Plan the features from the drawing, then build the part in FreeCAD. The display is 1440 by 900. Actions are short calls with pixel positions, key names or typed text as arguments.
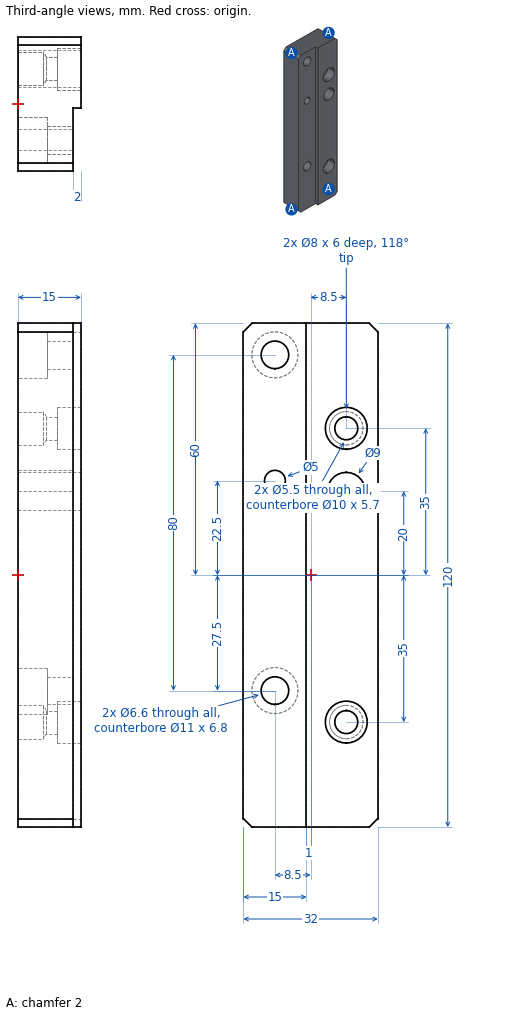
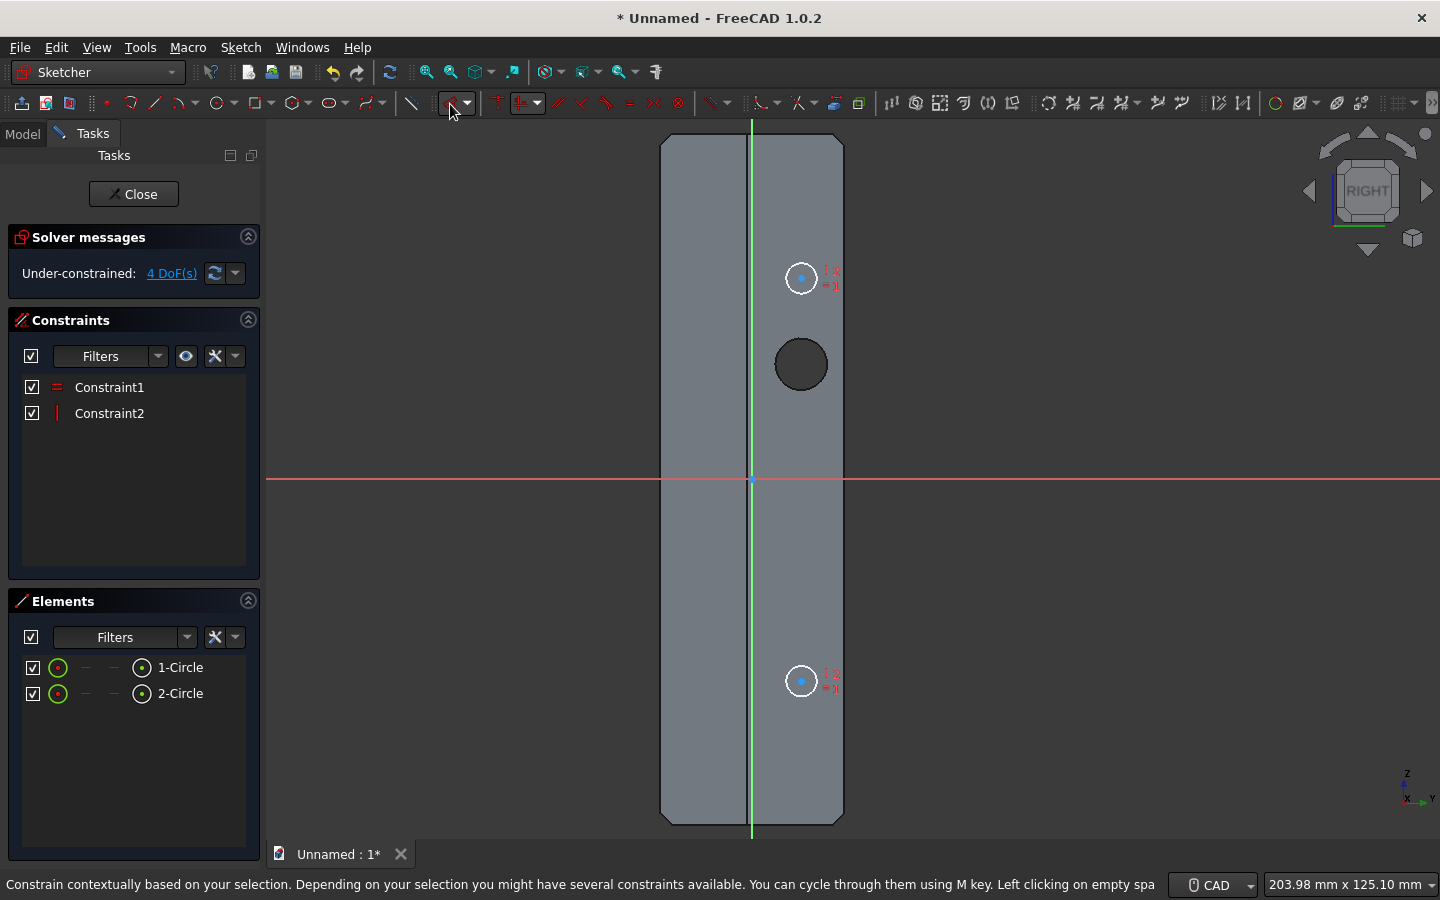
scroll(812, 268, up, 2)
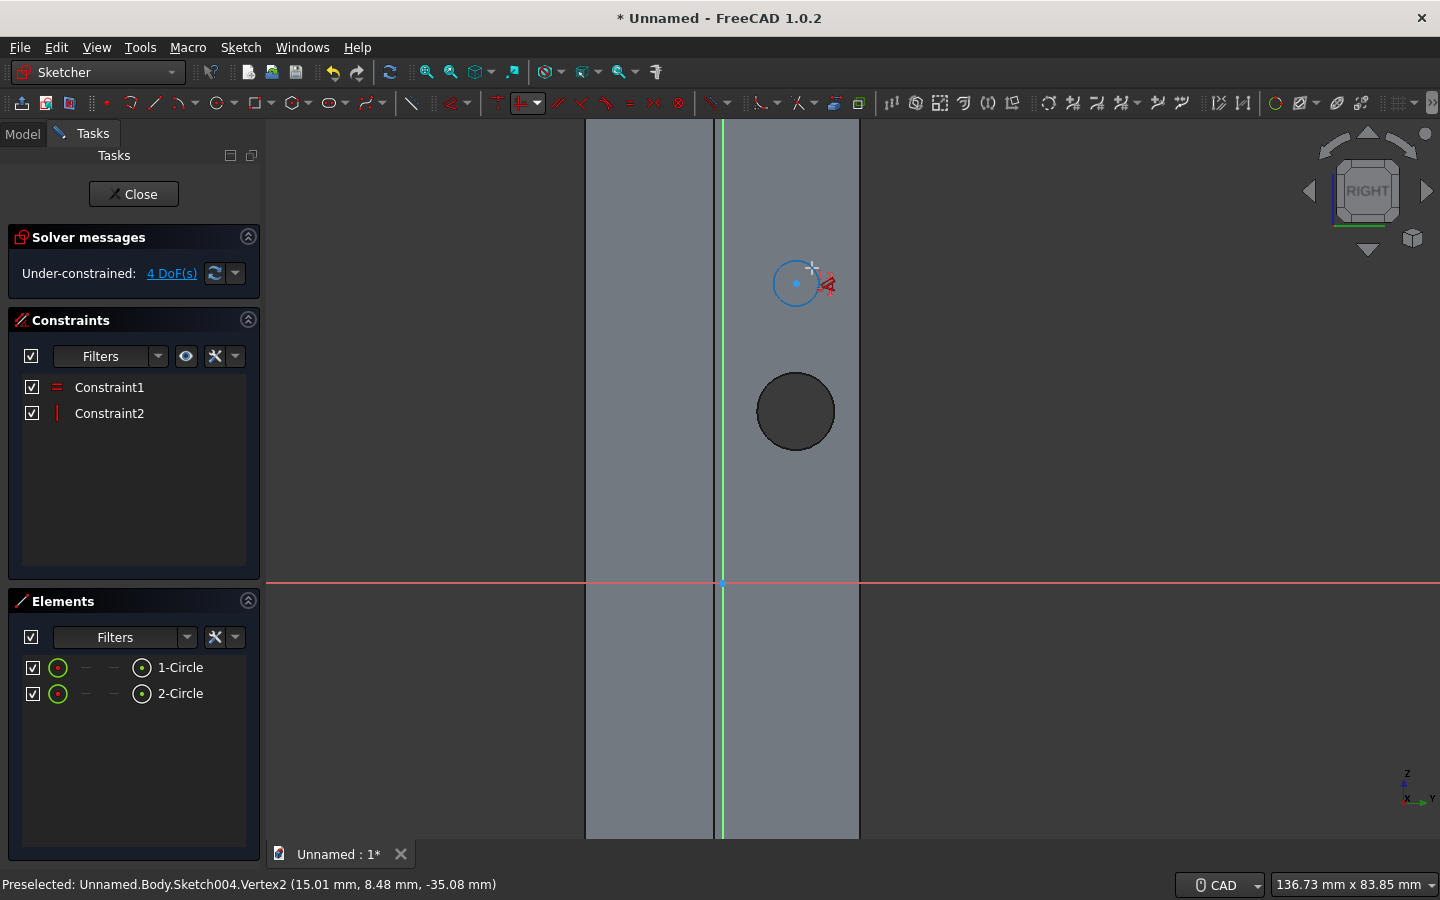
click(812, 267)
click(834, 244)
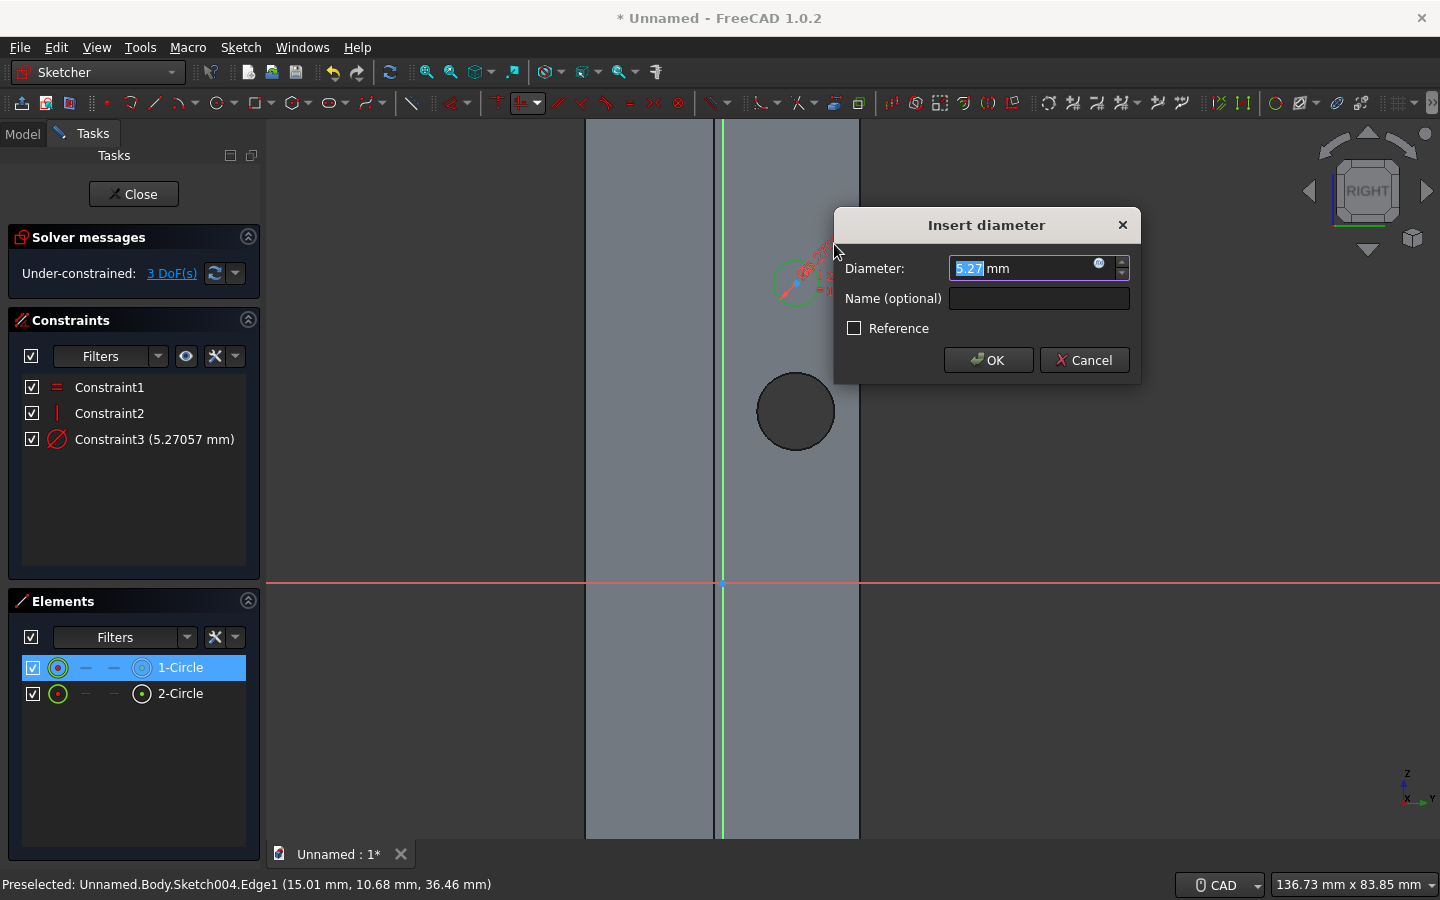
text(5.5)
key(Return)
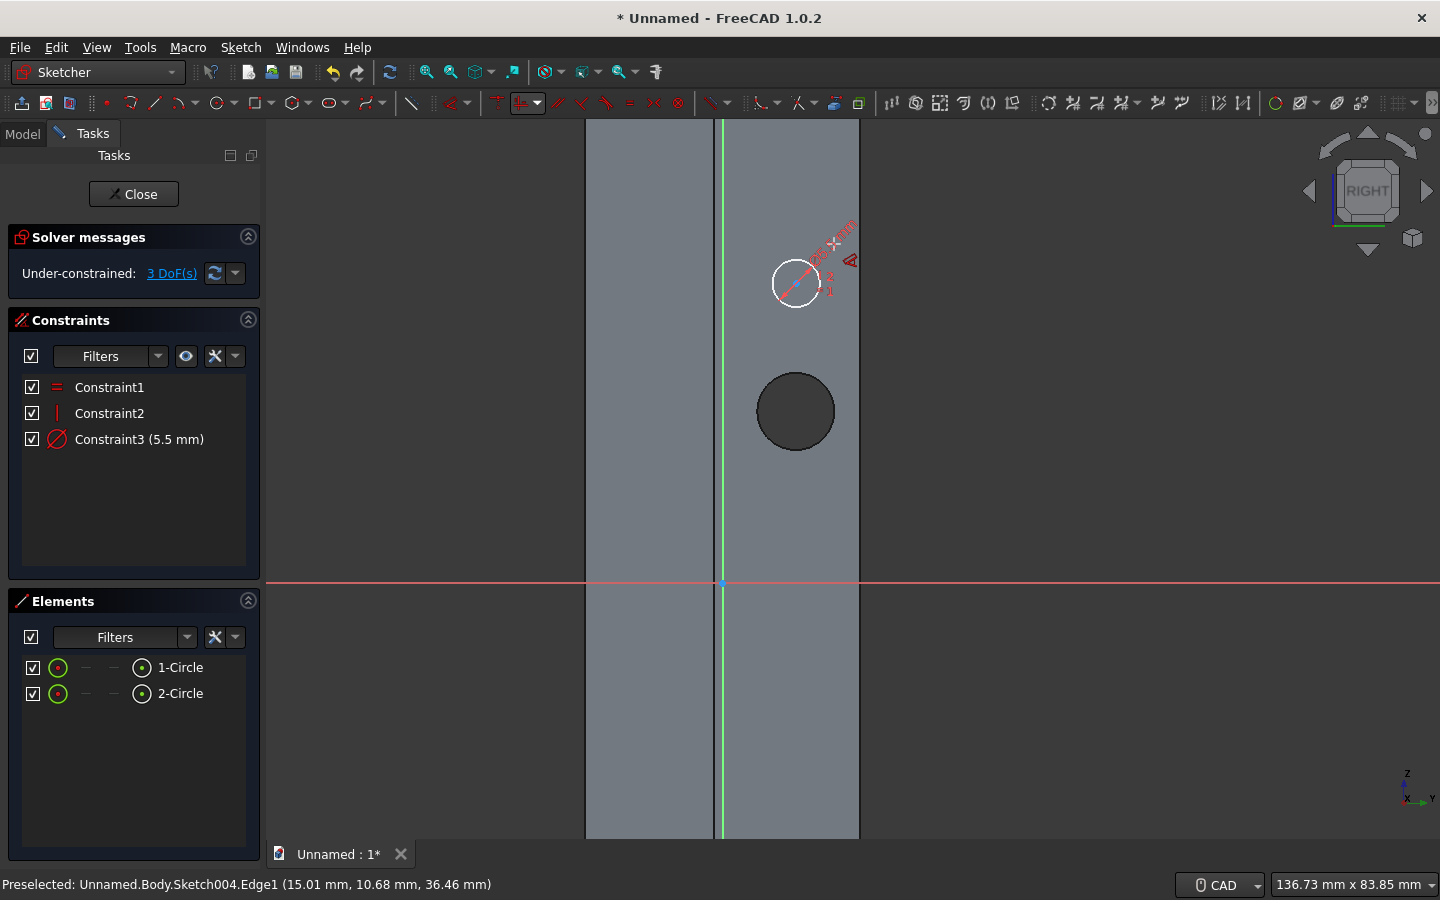
click(796, 283)
click(689, 433)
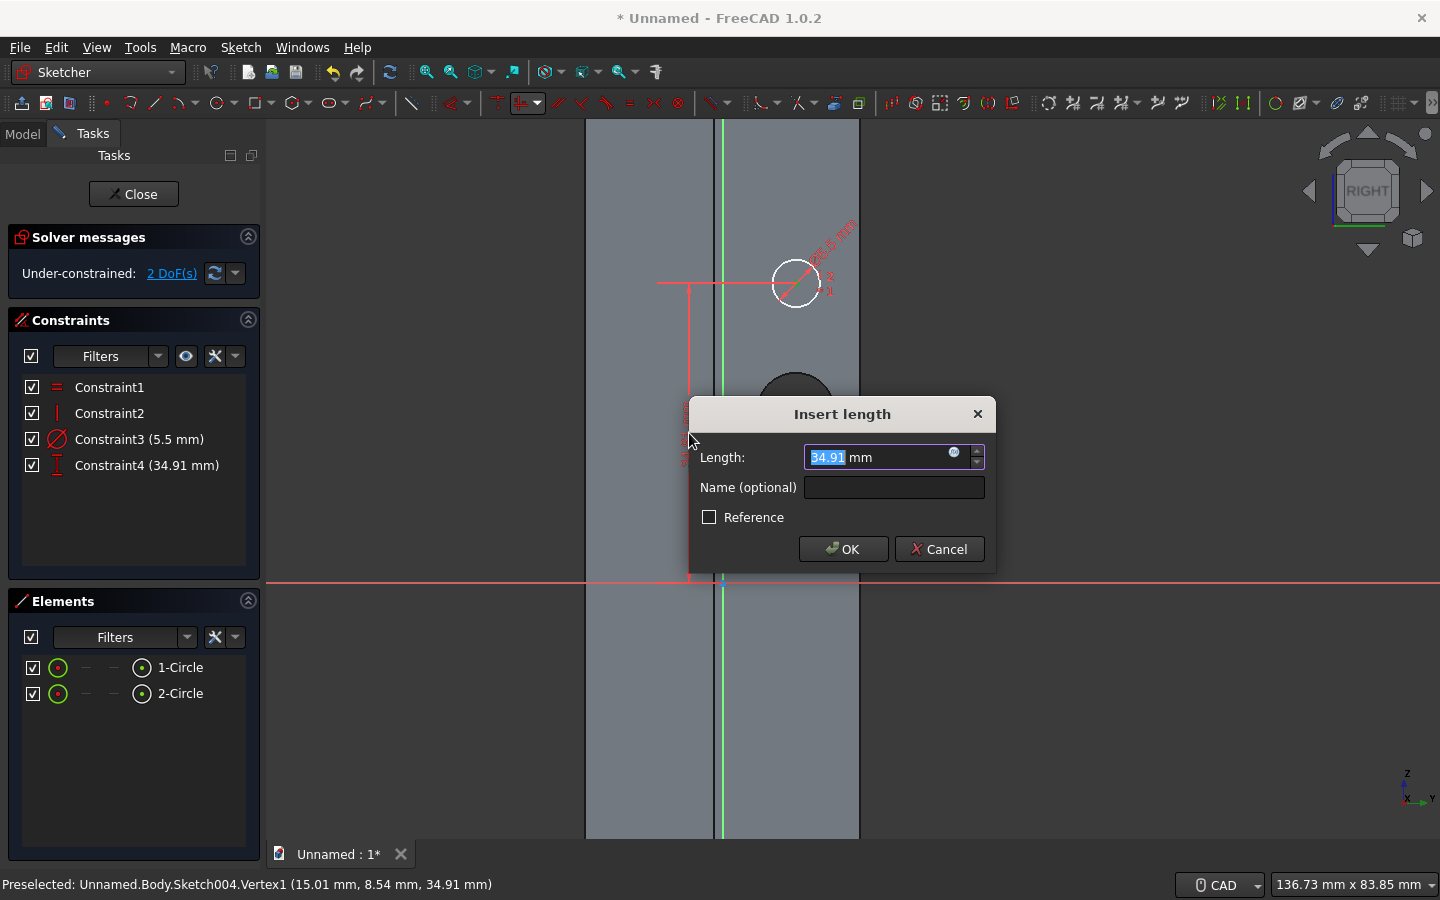
text(35)
key(Return)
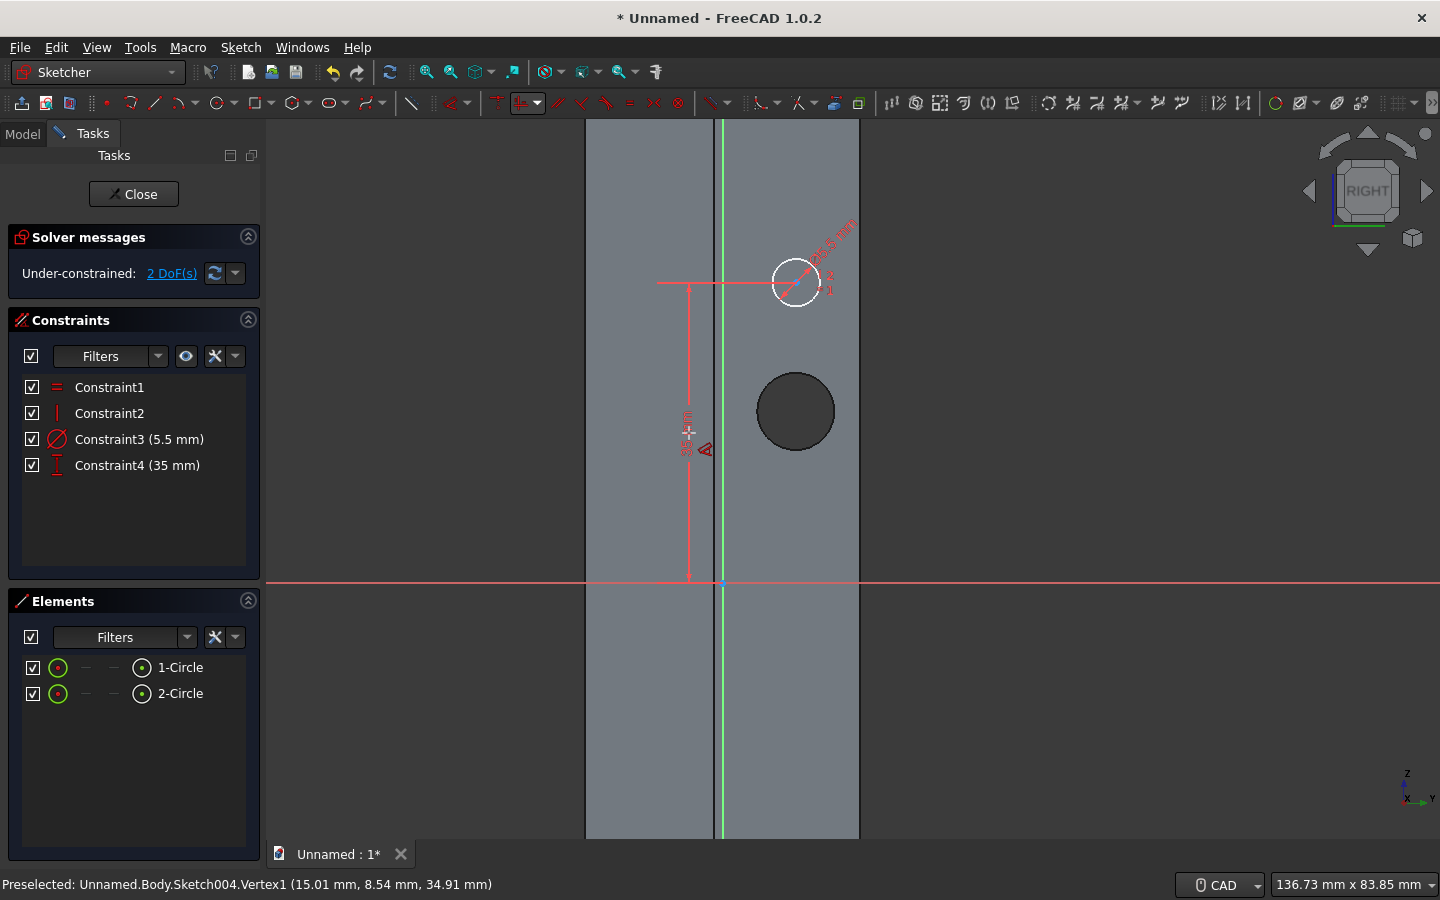
scroll(812, 267, down, 2)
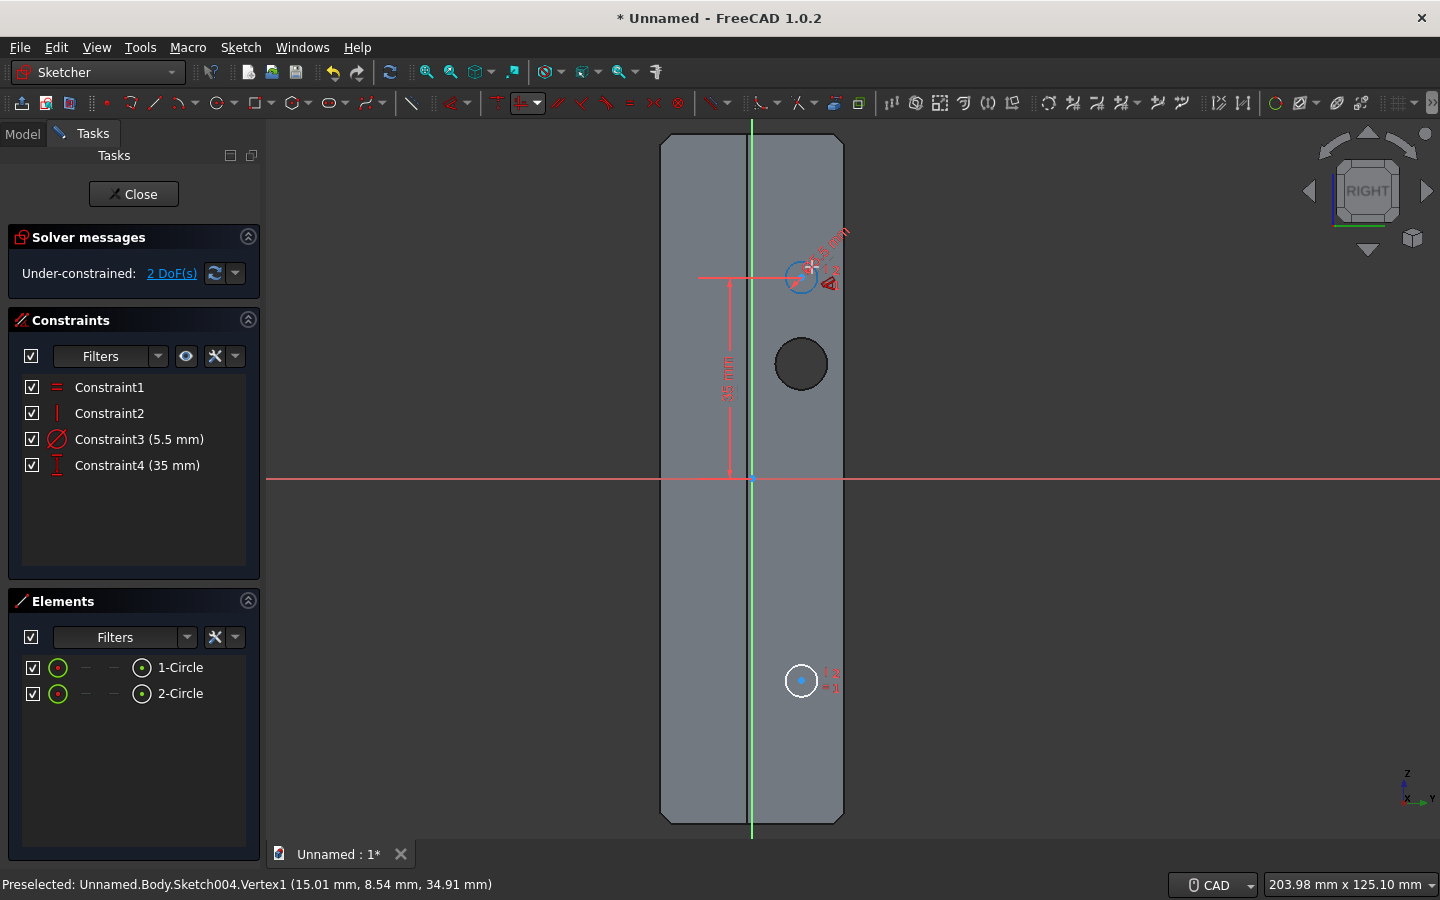
click(802, 681)
click(718, 580)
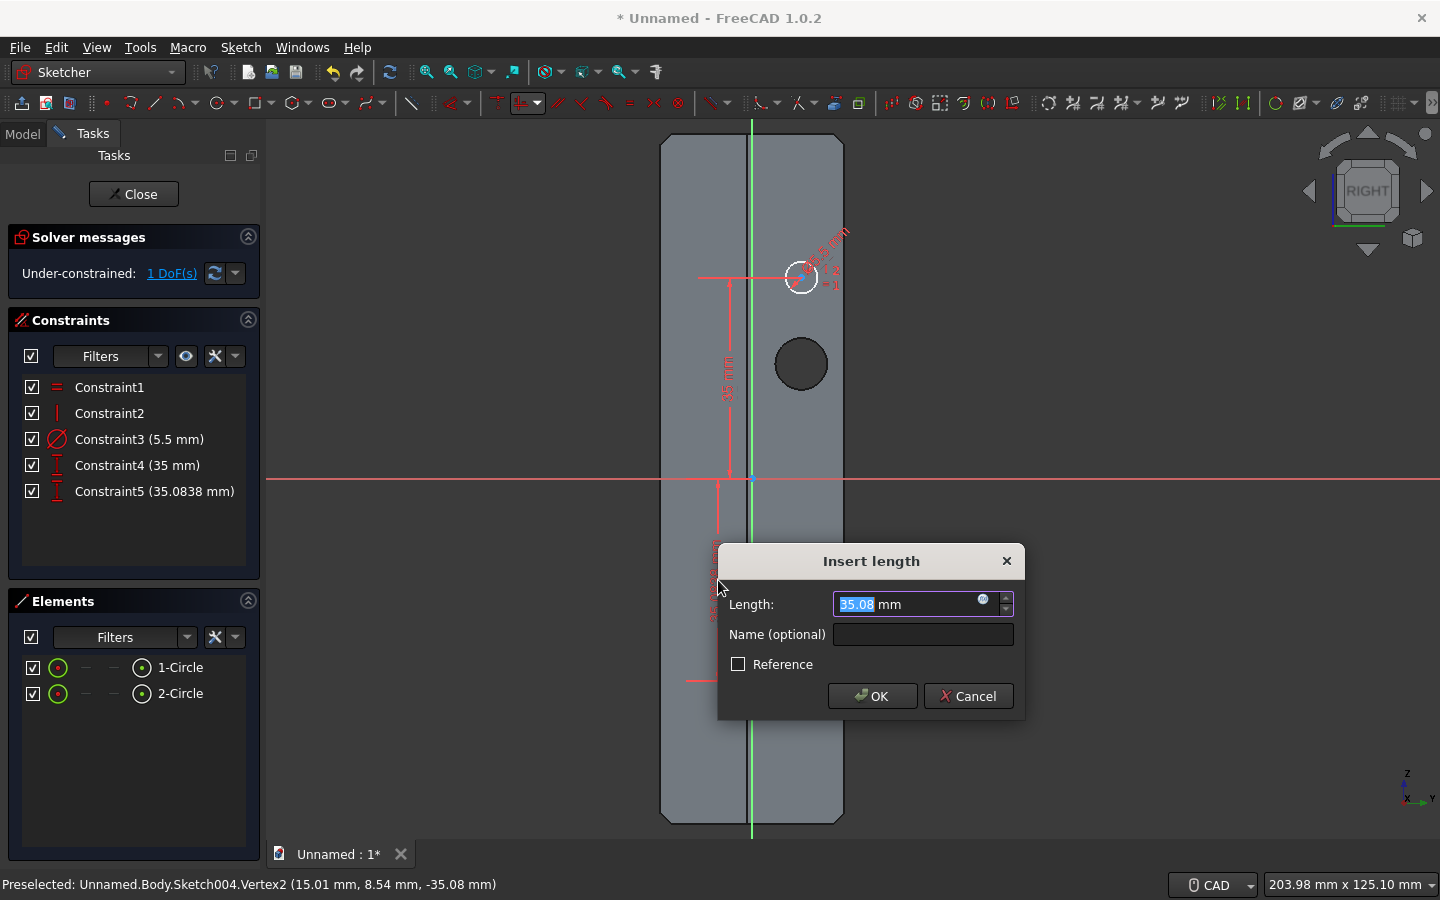
text(35)
key(Return)